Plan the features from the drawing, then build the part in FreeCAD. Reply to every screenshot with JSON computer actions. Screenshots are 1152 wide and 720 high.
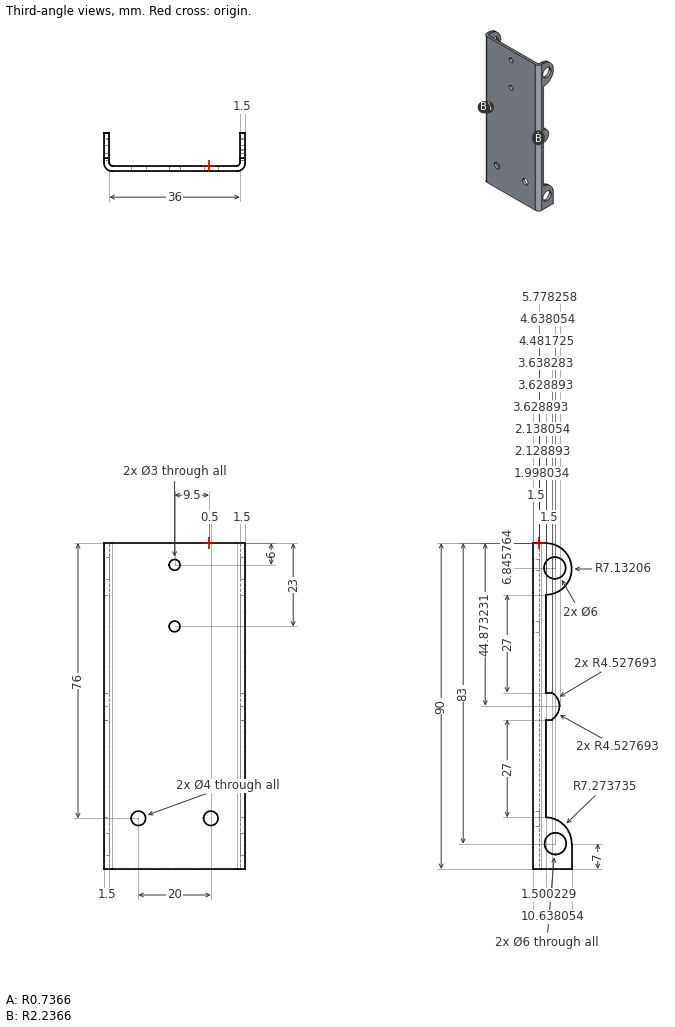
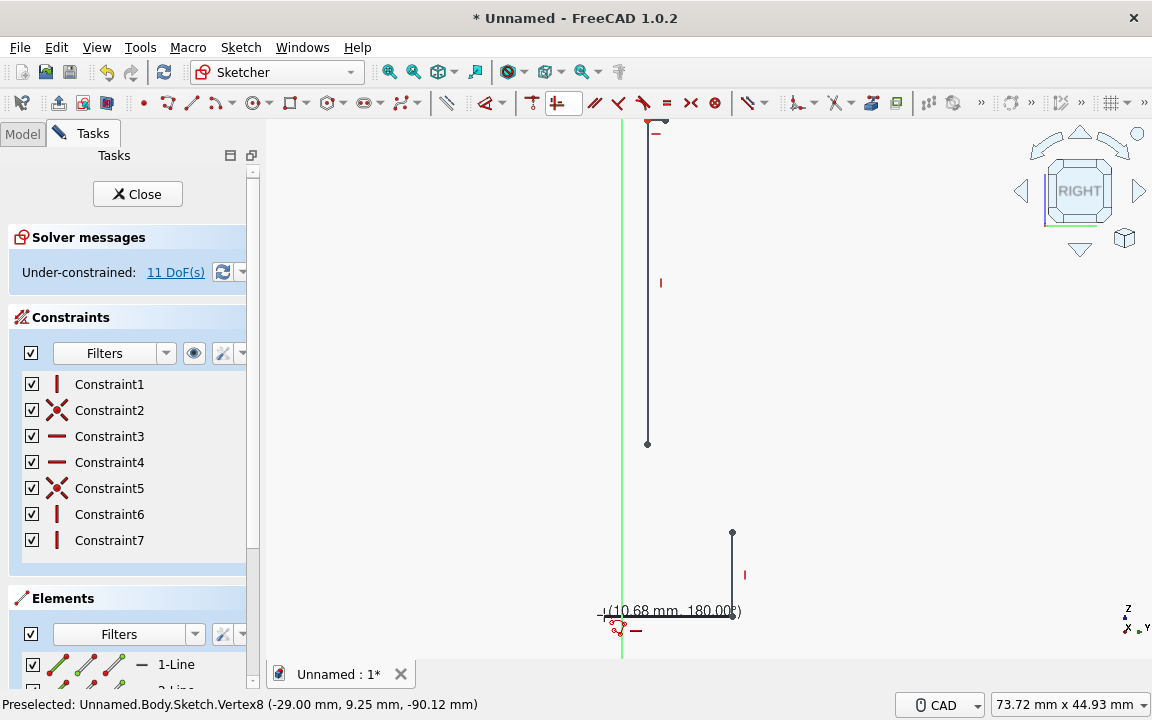
{"action": "left_click", "coordinate": [604, 615]}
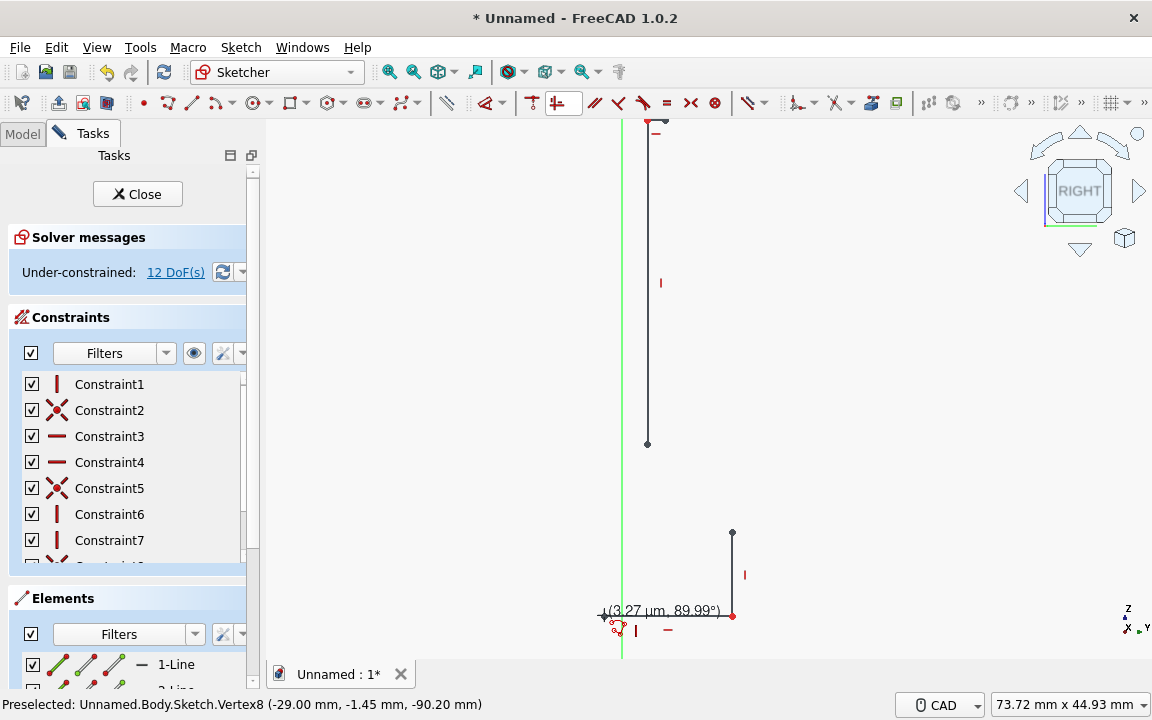
{"action": "scroll", "coordinate": [629, 525], "scroll_direction": "down", "scroll_amount": 6}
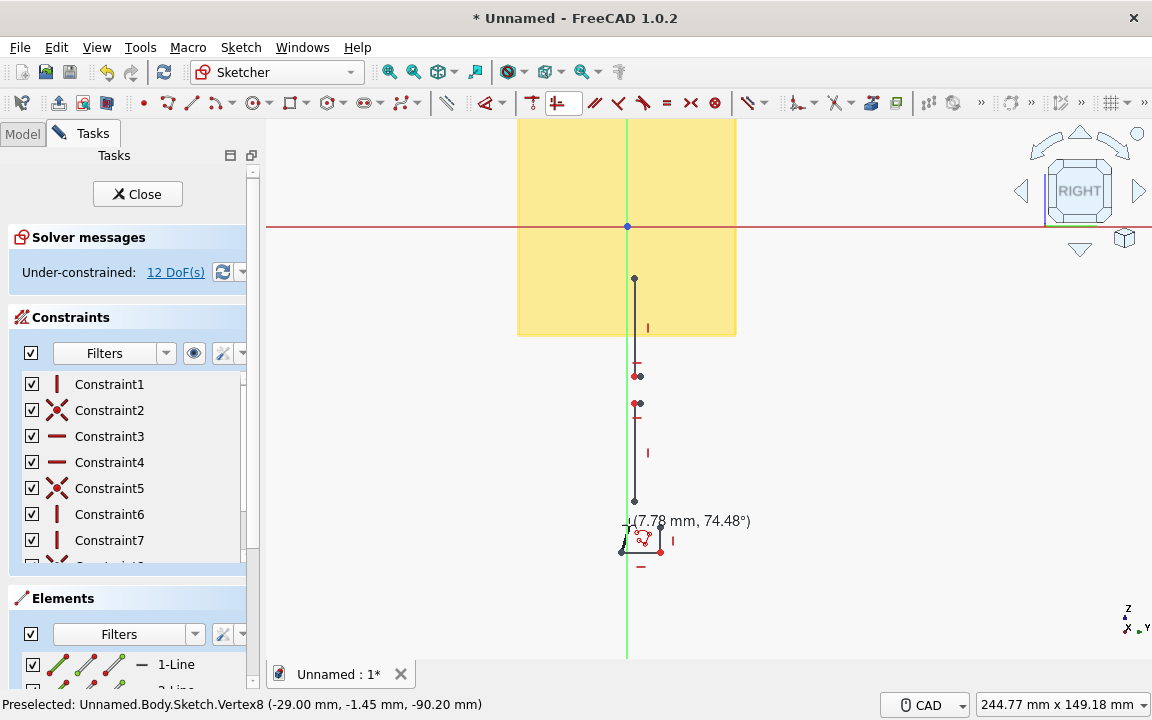
{"action": "scroll", "coordinate": [622, 227], "scroll_direction": "up", "scroll_amount": 6}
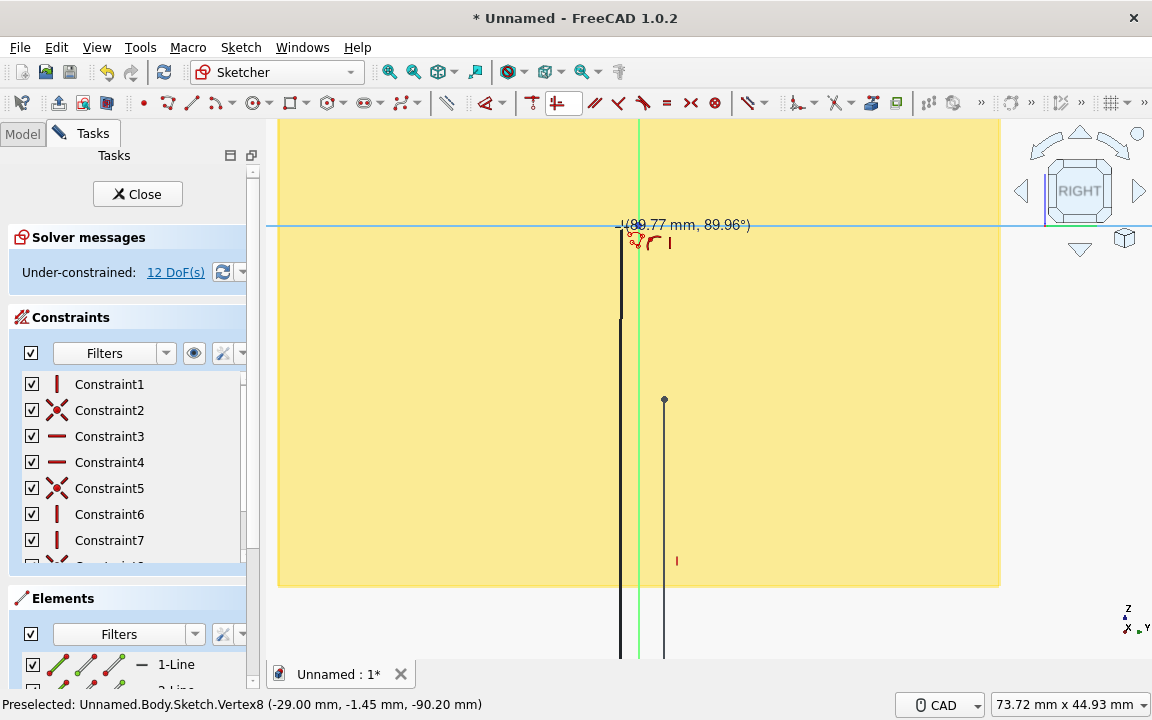
{"action": "left_click", "coordinate": [620, 226]}
{"action": "left_click", "coordinate": [664, 235]}
{"action": "right_click", "coordinate": [664, 235]}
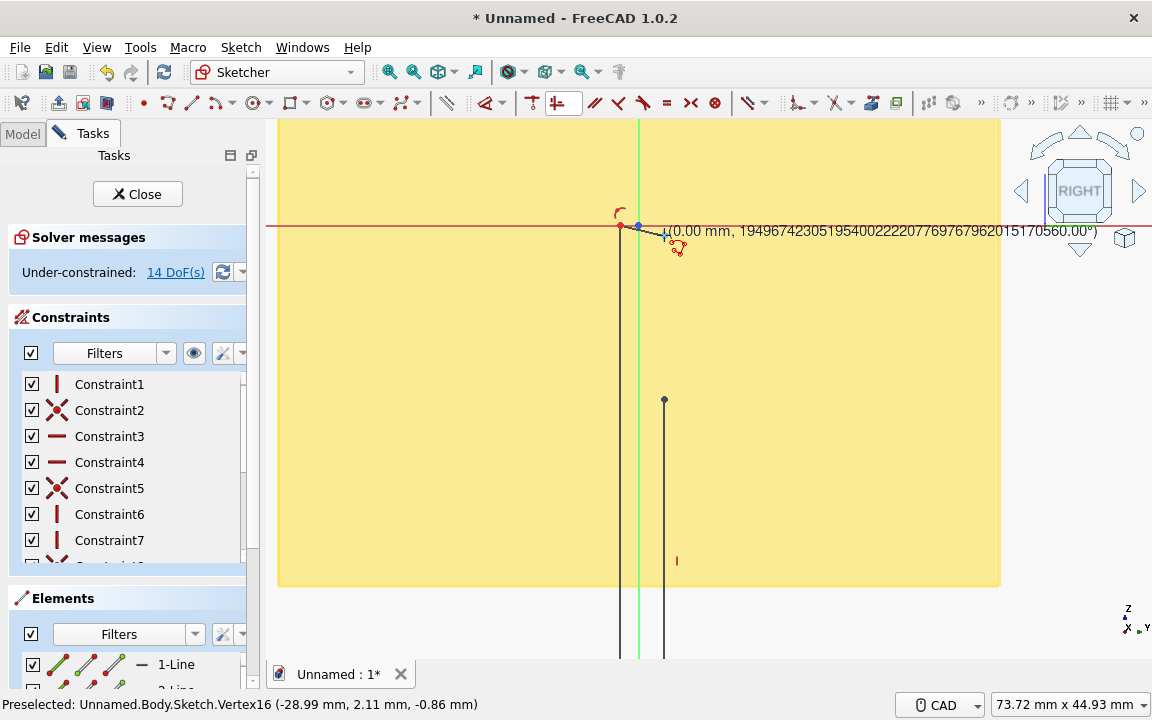
{"action": "left_click", "coordinate": [234, 104]}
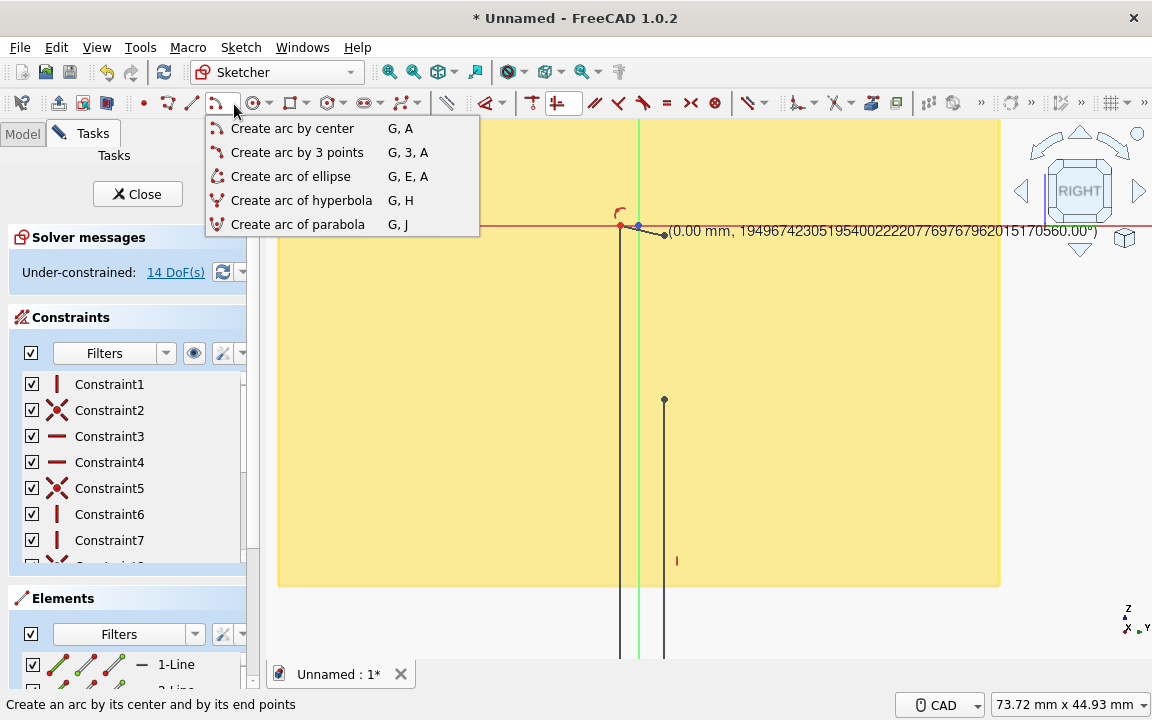
{"action": "left_click", "coordinate": [342, 152]}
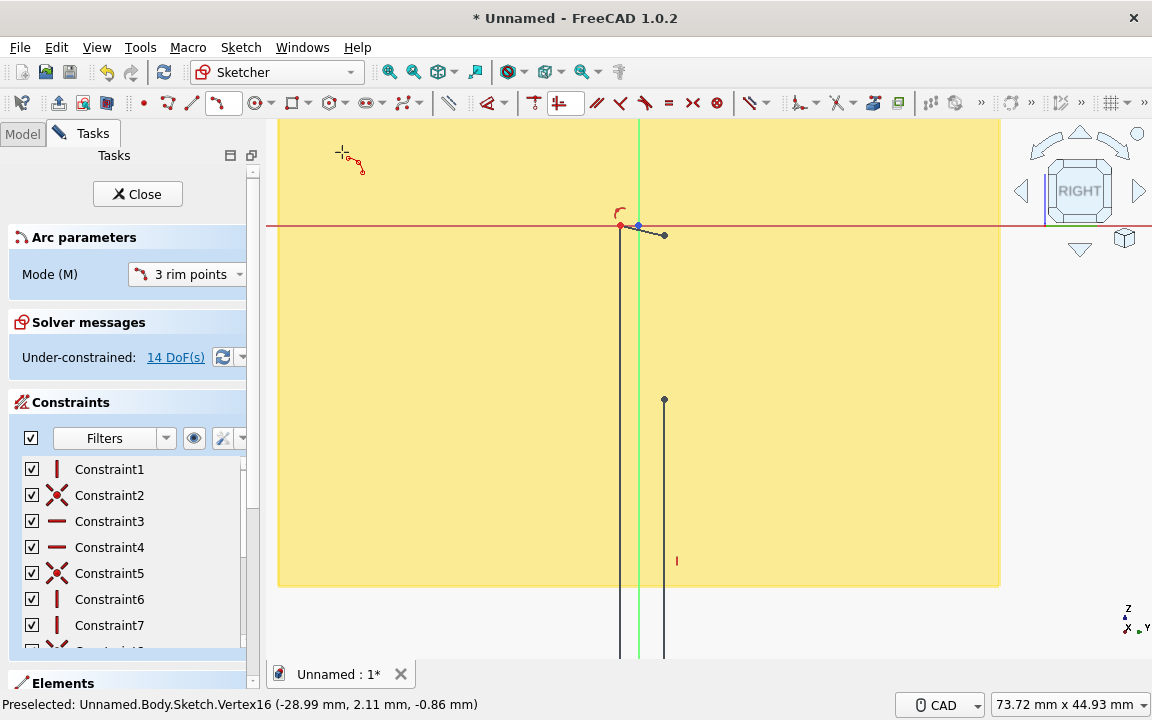
{"action": "scroll", "coordinate": [621, 226], "scroll_direction": "down", "scroll_amount": 6}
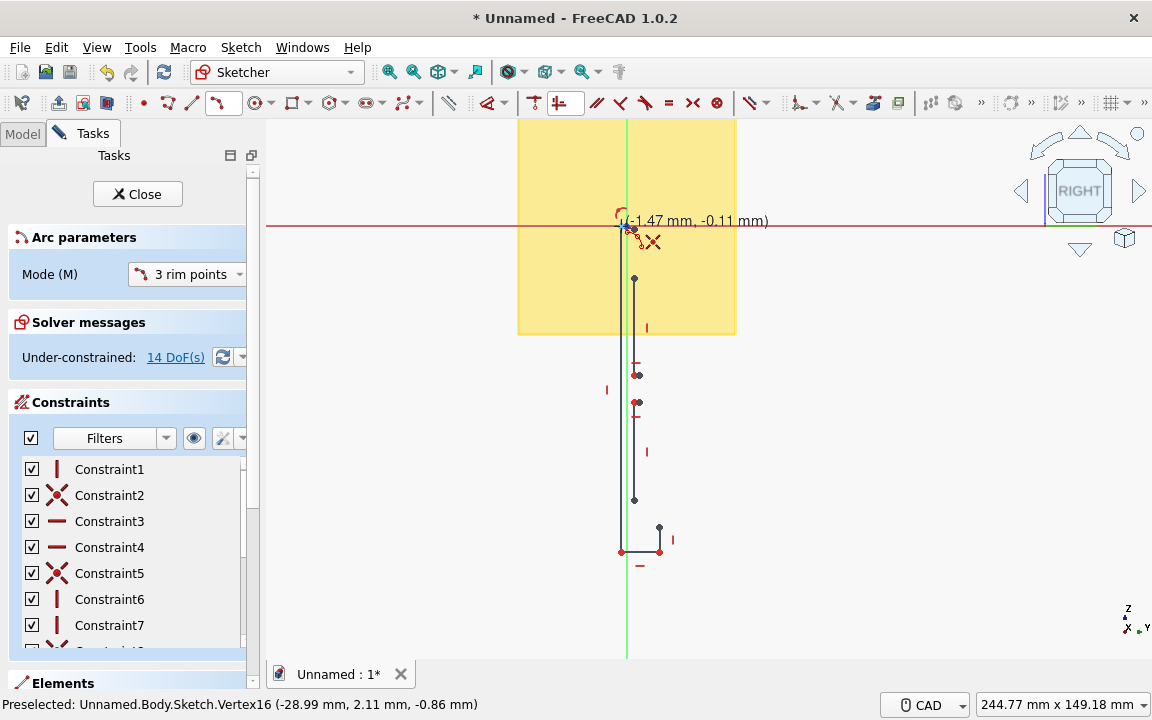
{"action": "scroll", "coordinate": [640, 375], "scroll_direction": "up", "scroll_amount": 9}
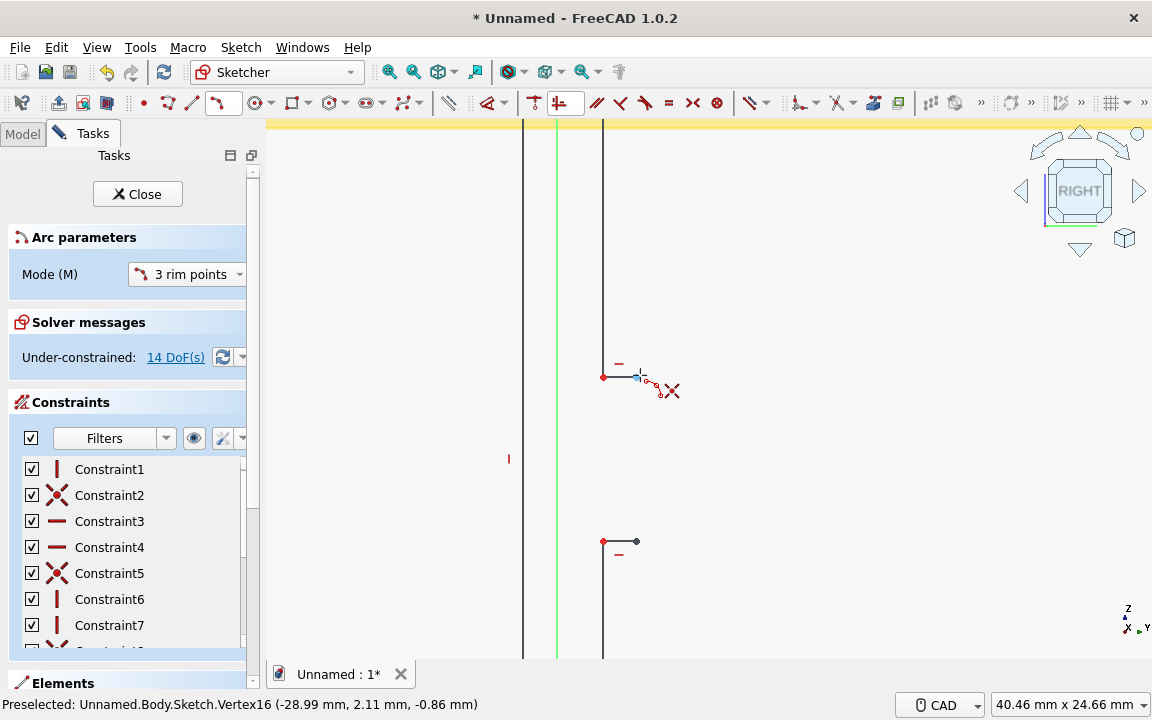
{"action": "left_click", "coordinate": [636, 377]}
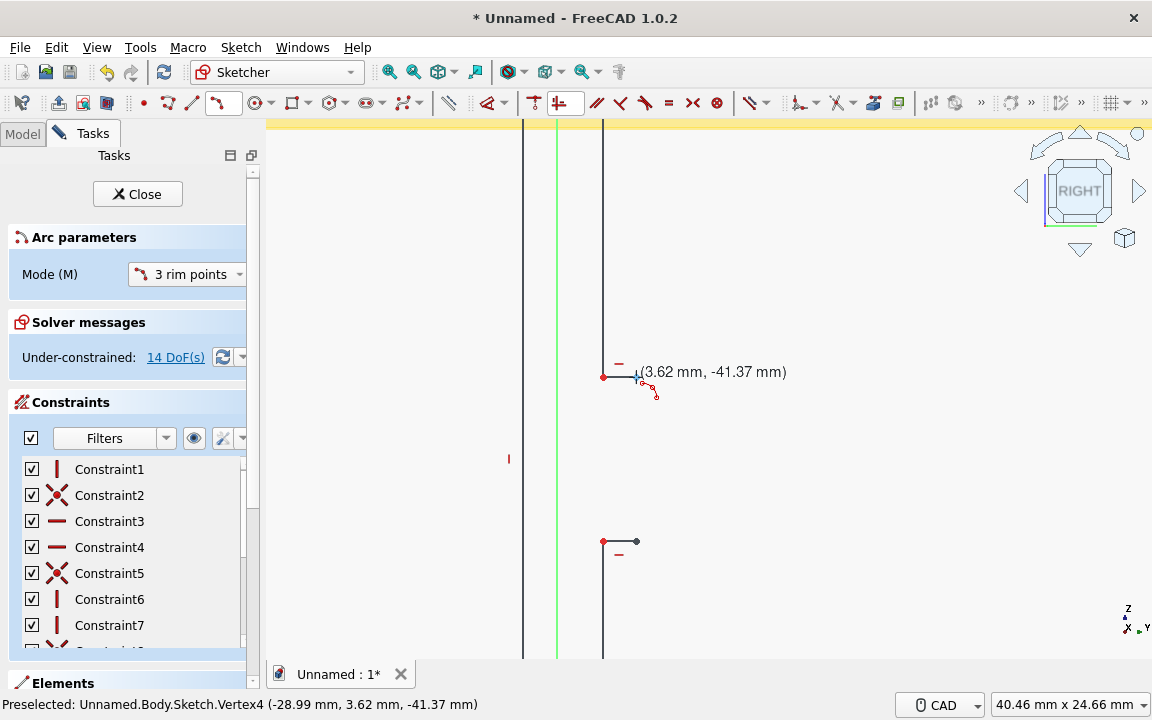
{"action": "scroll", "coordinate": [641, 376], "scroll_direction": "down", "scroll_amount": 9}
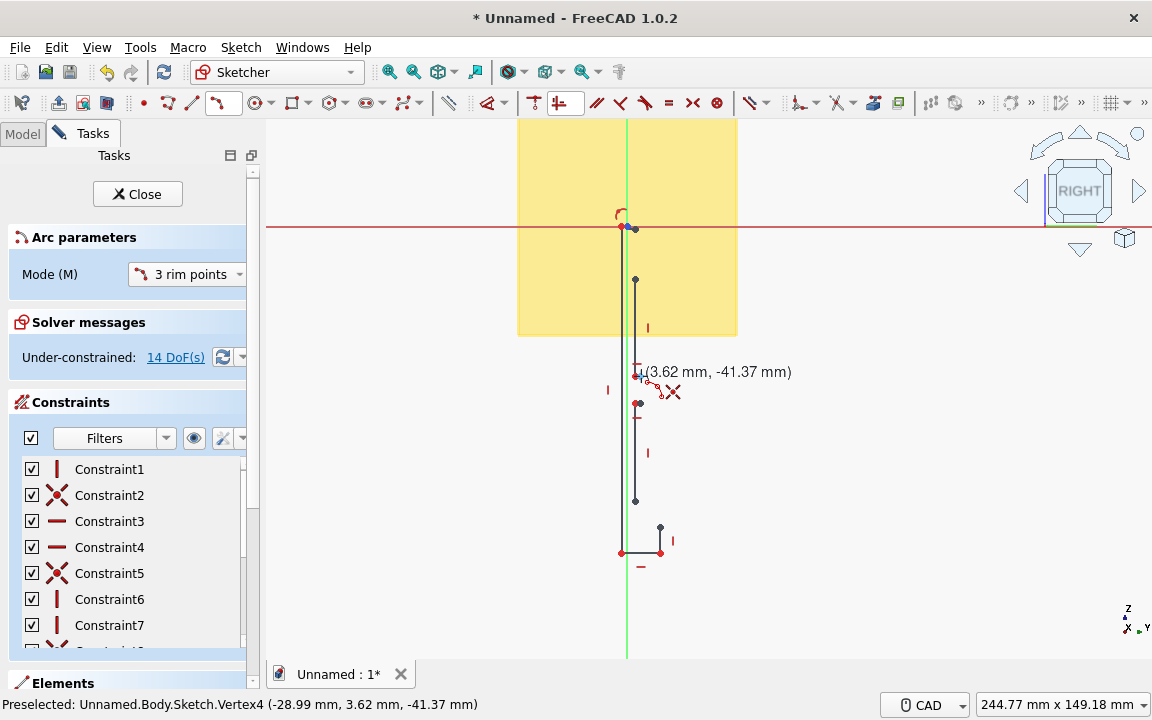
{"action": "left_click", "coordinate": [648, 389]}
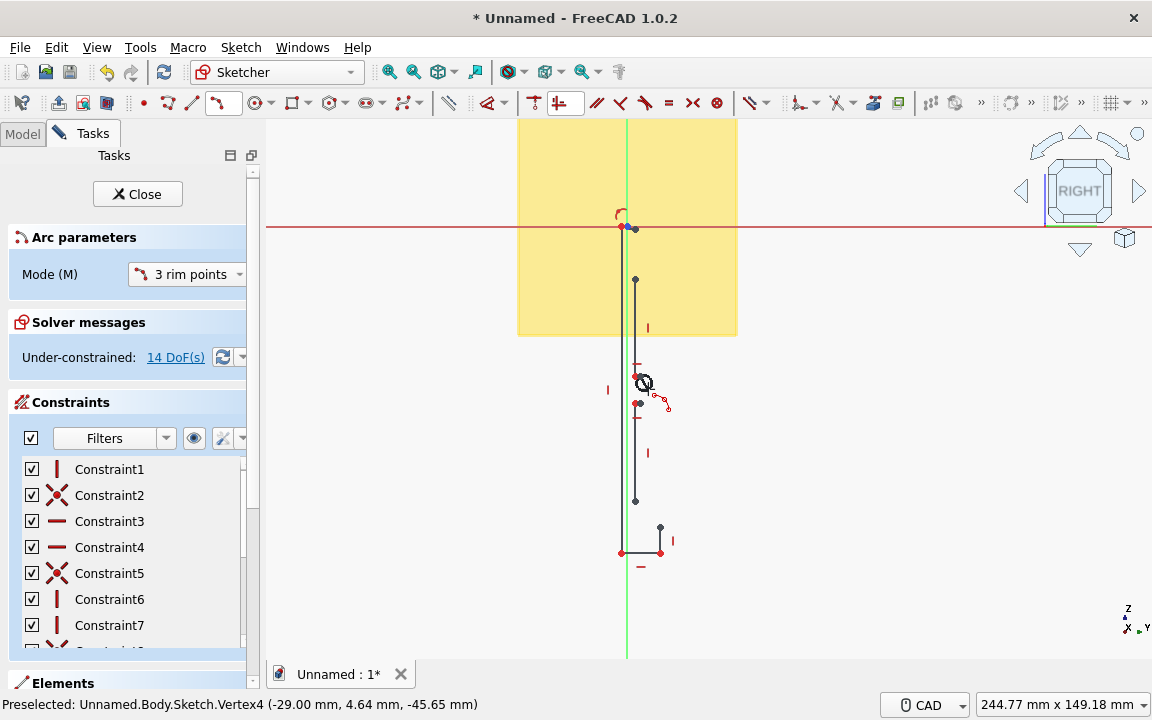
{"action": "scroll", "coordinate": [646, 382], "scroll_direction": "up", "scroll_amount": 11}